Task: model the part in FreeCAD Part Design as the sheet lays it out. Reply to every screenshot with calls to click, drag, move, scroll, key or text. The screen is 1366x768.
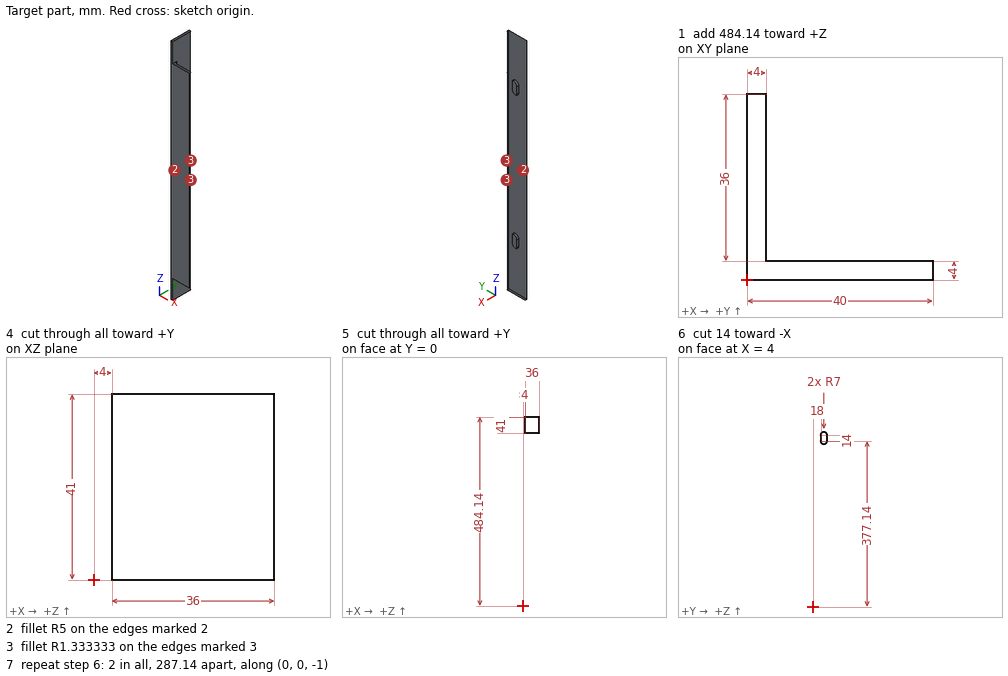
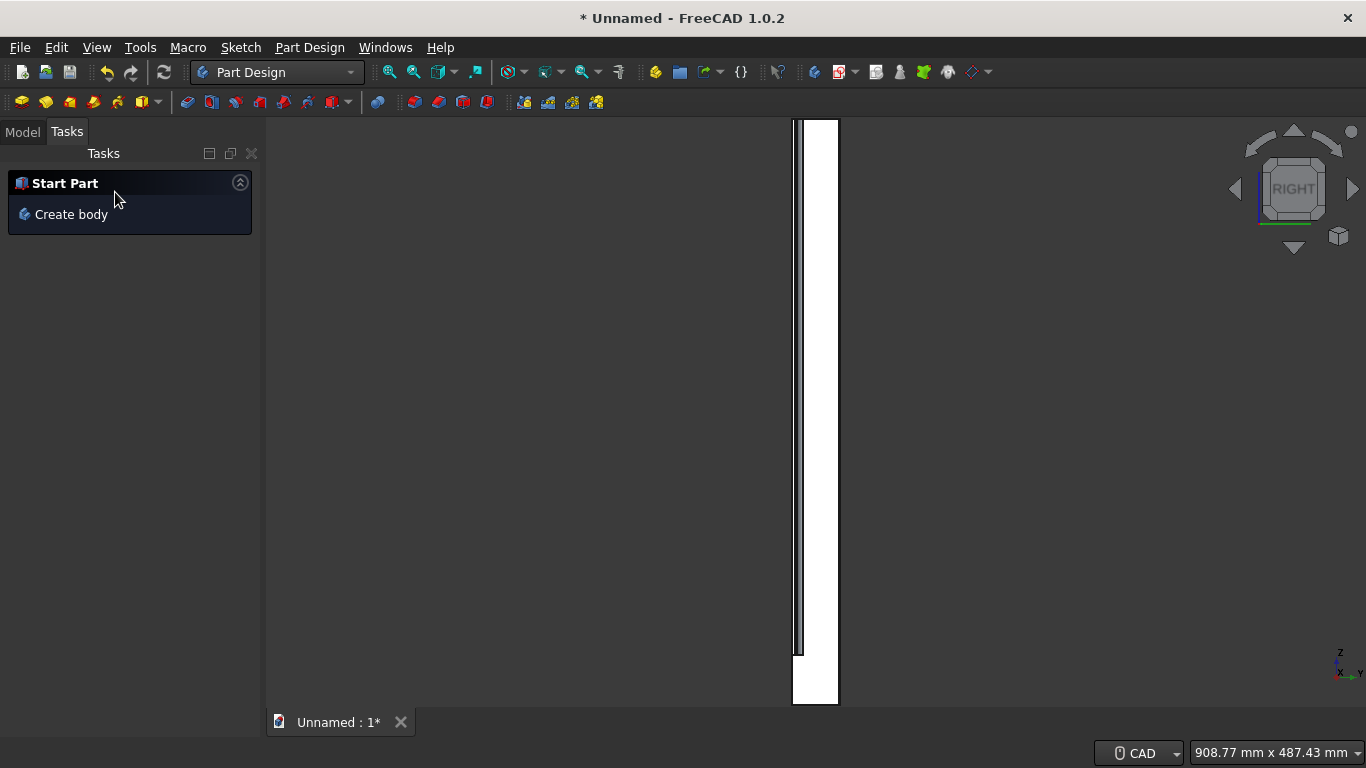
key(0)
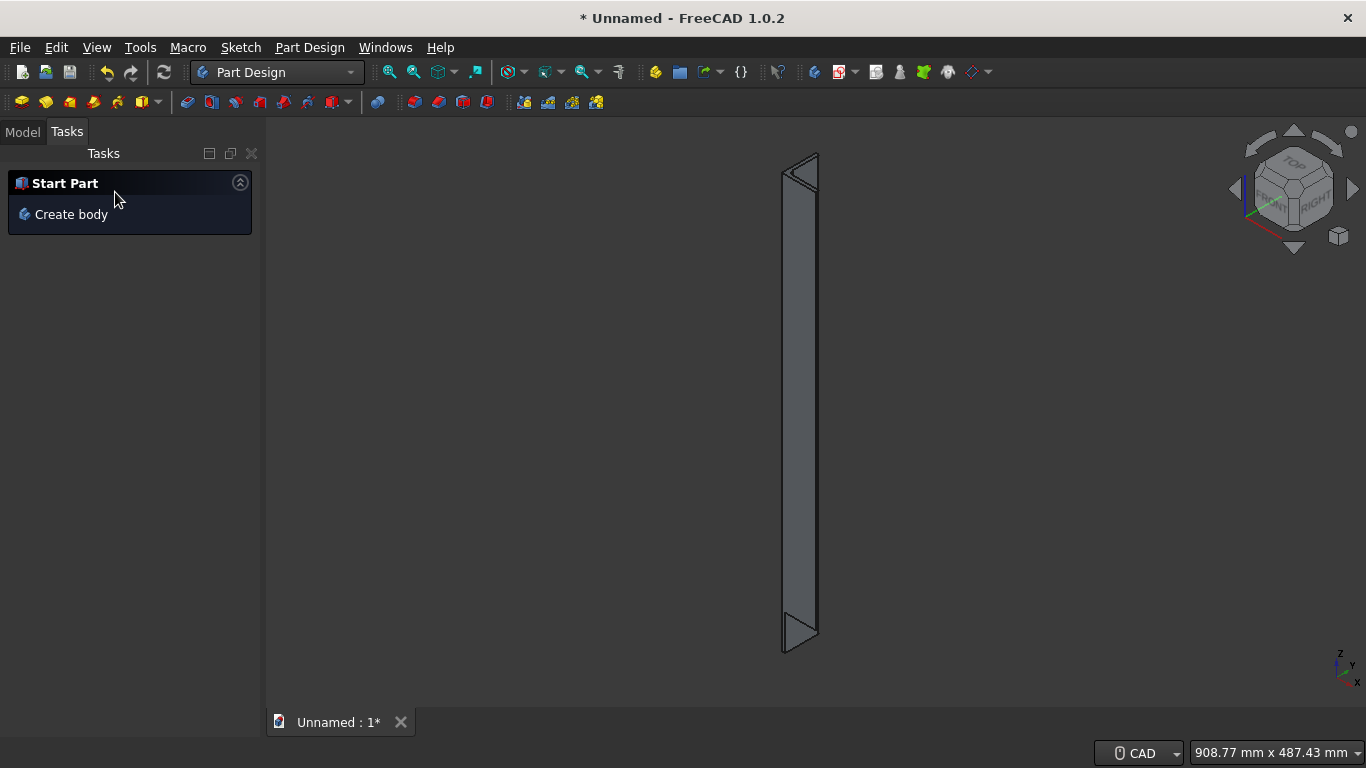
click(799, 216)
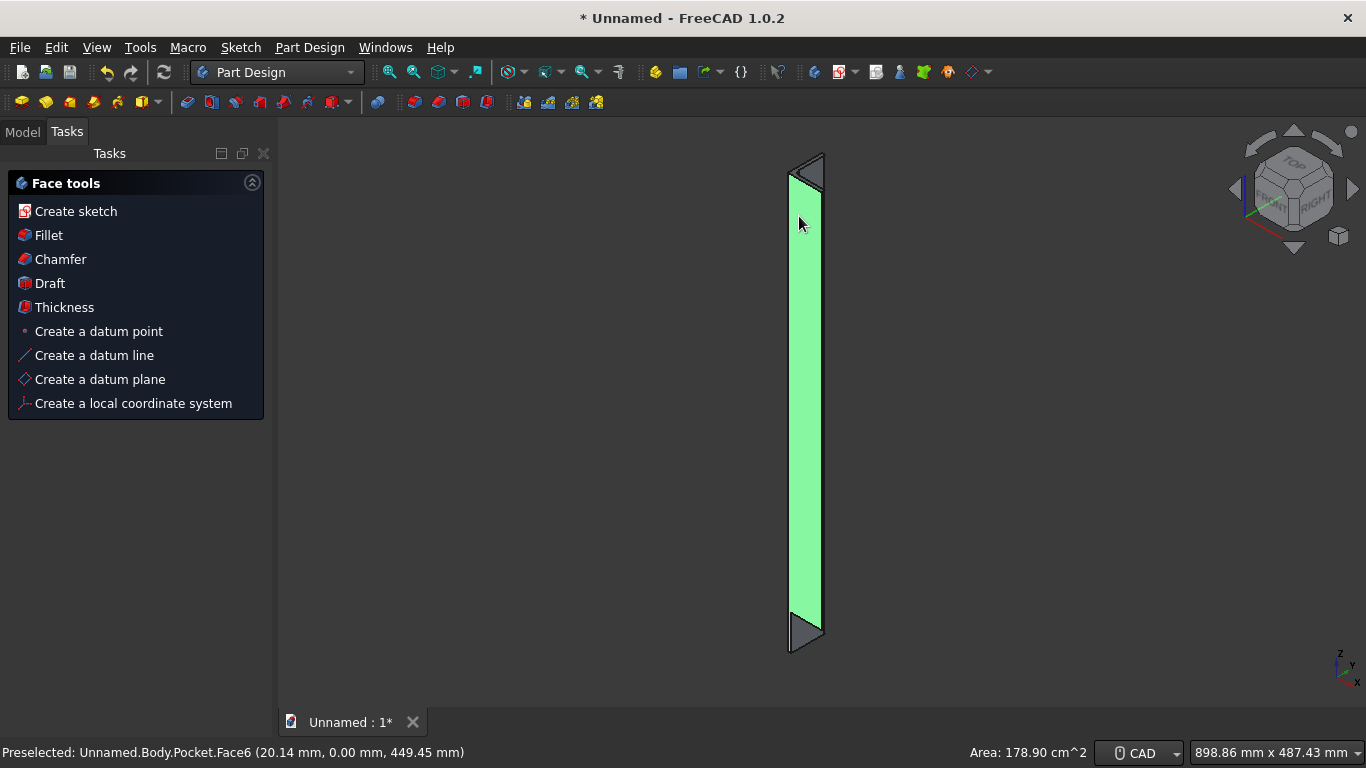
click(840, 72)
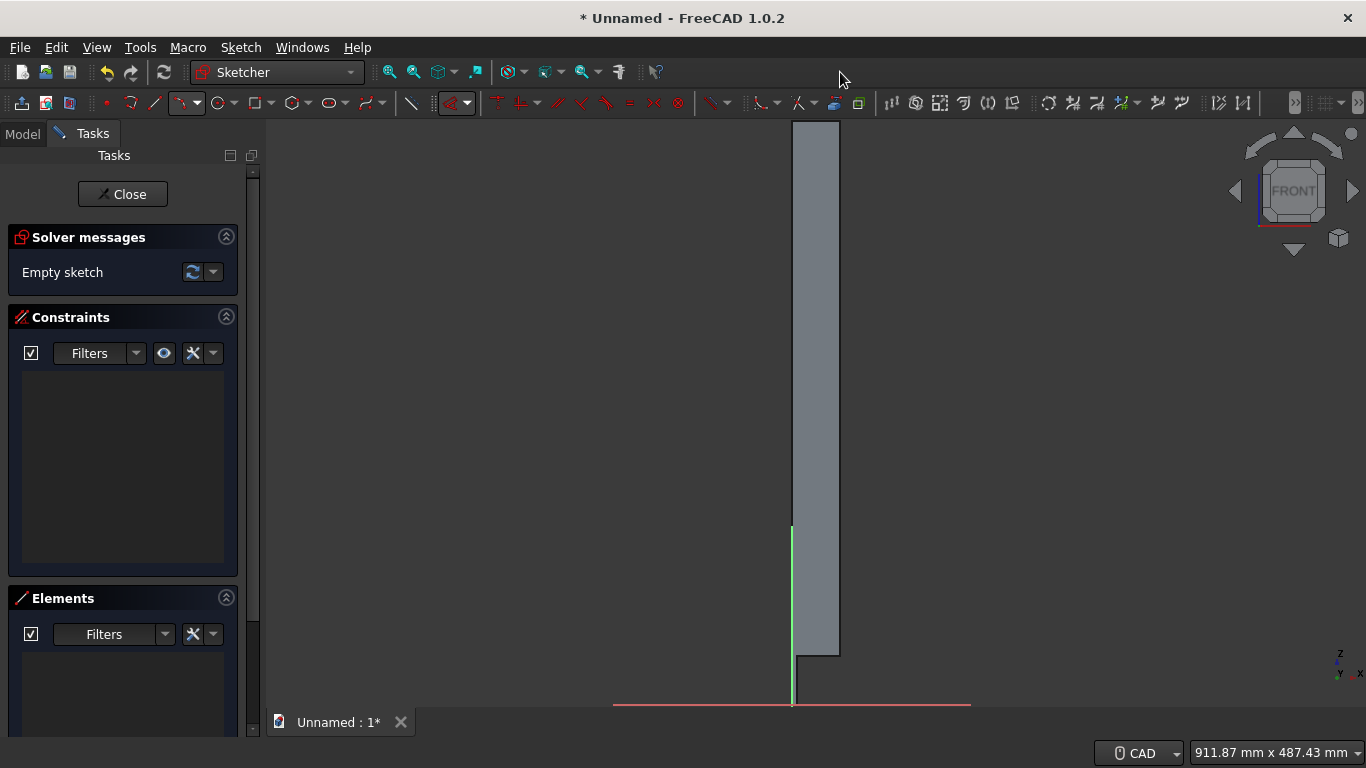
scroll(748, 413, down, 5)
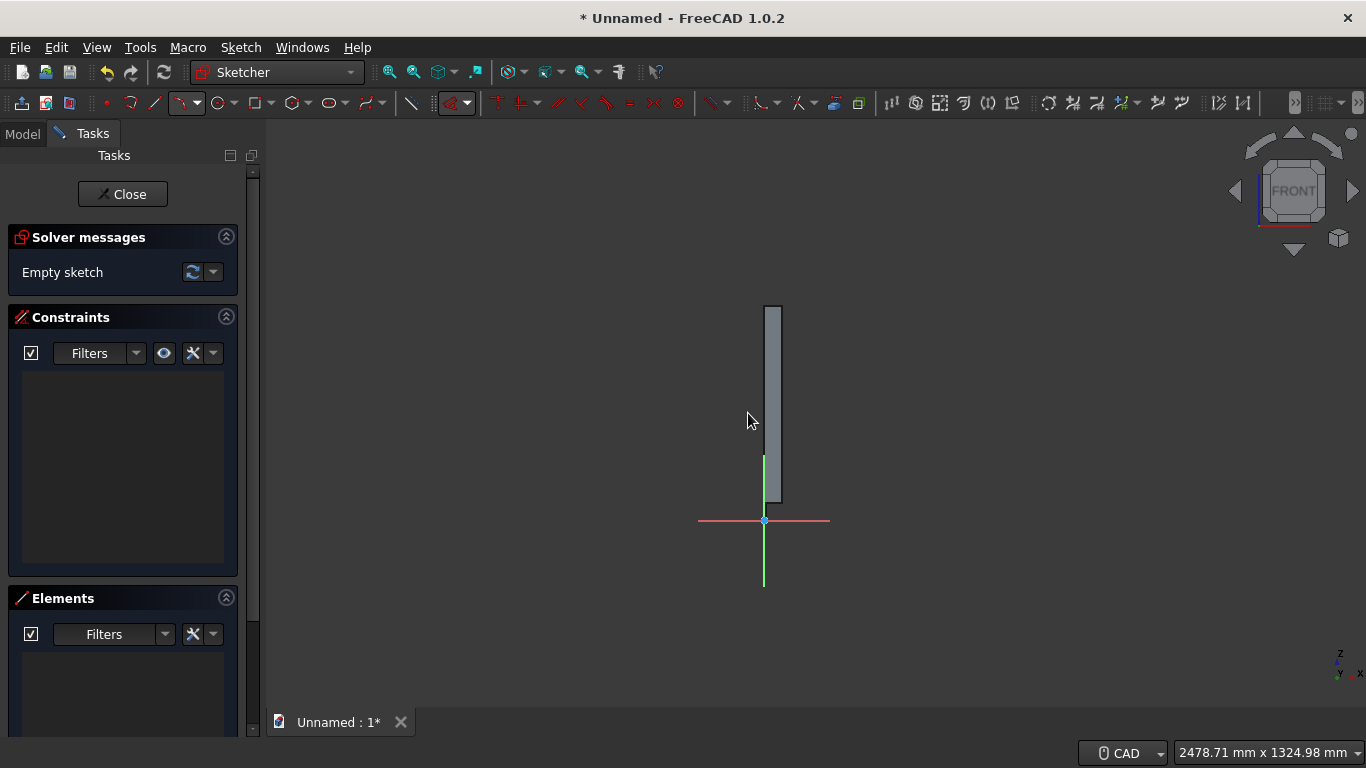
scroll(776, 310, up, 15)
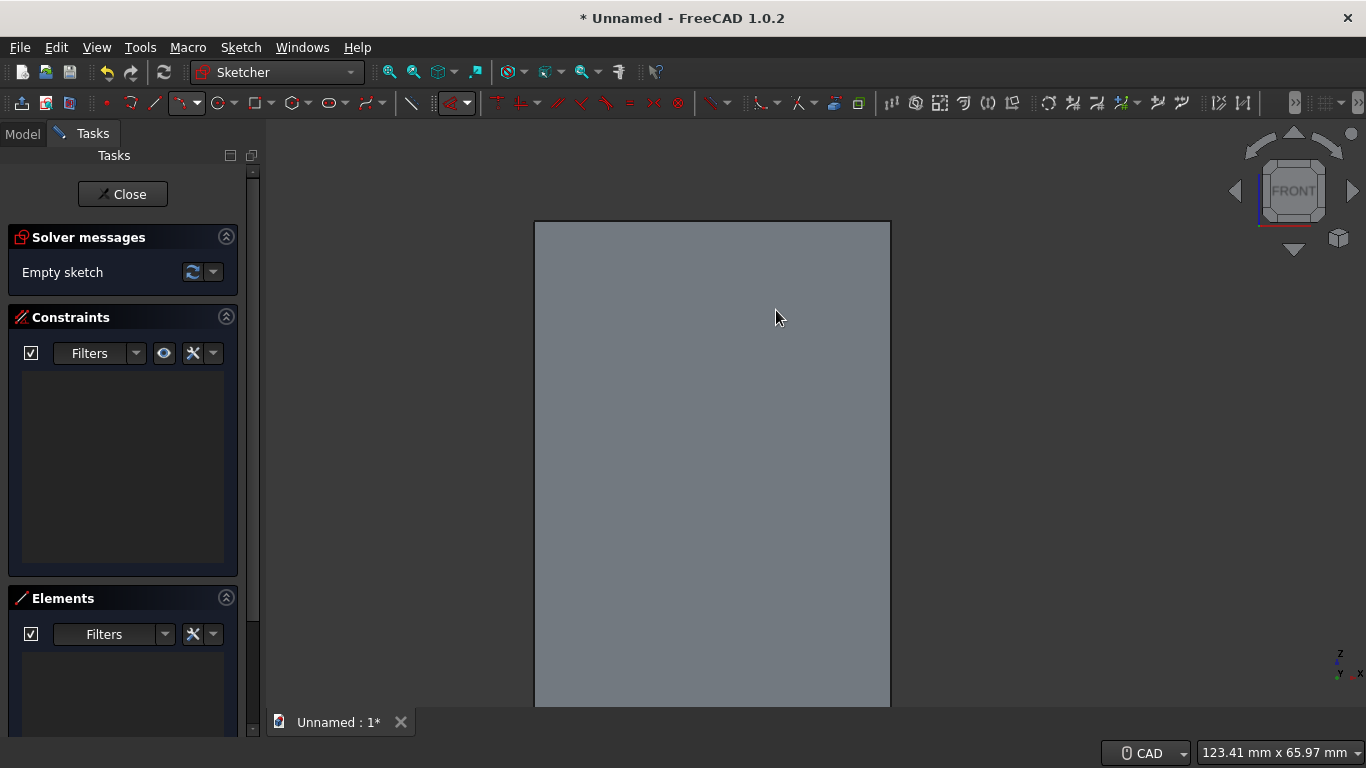
click(256, 104)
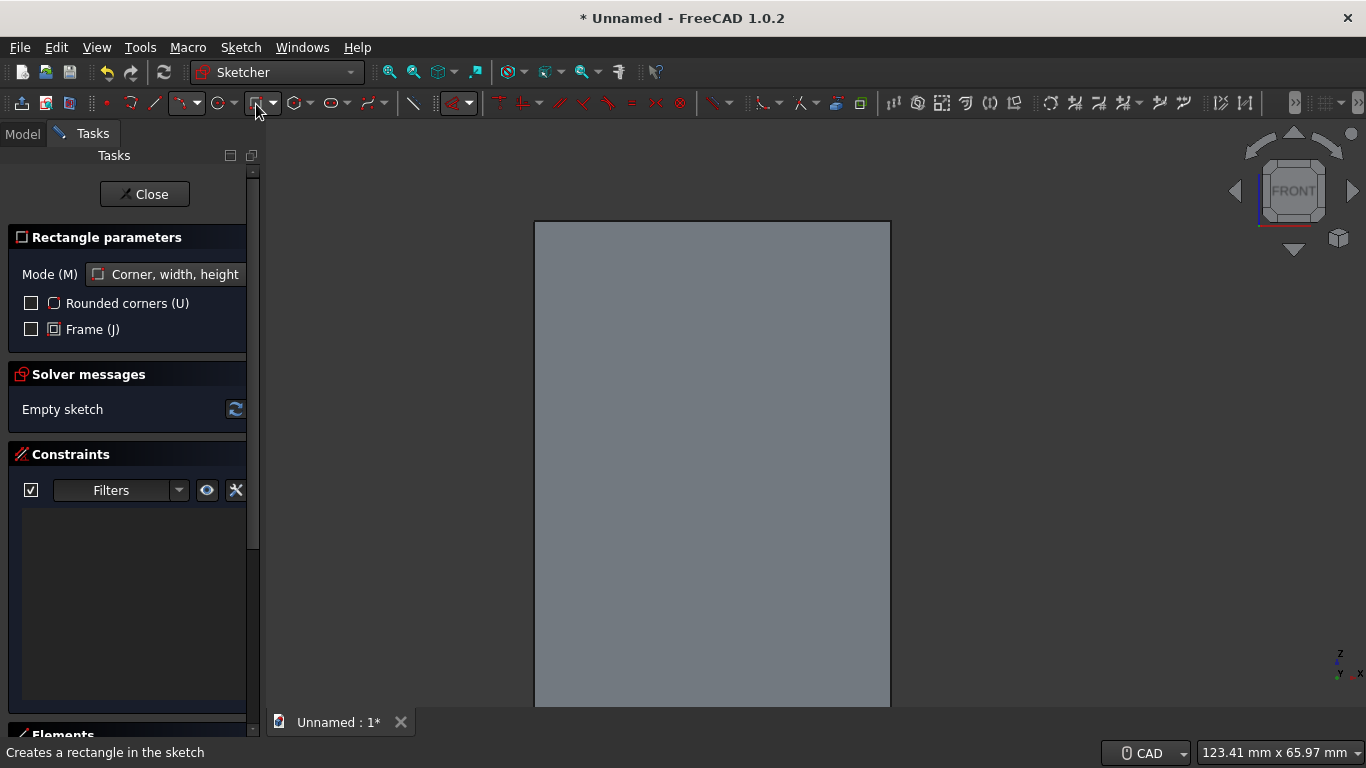
click(570, 221)
click(891, 587)
key(Escape)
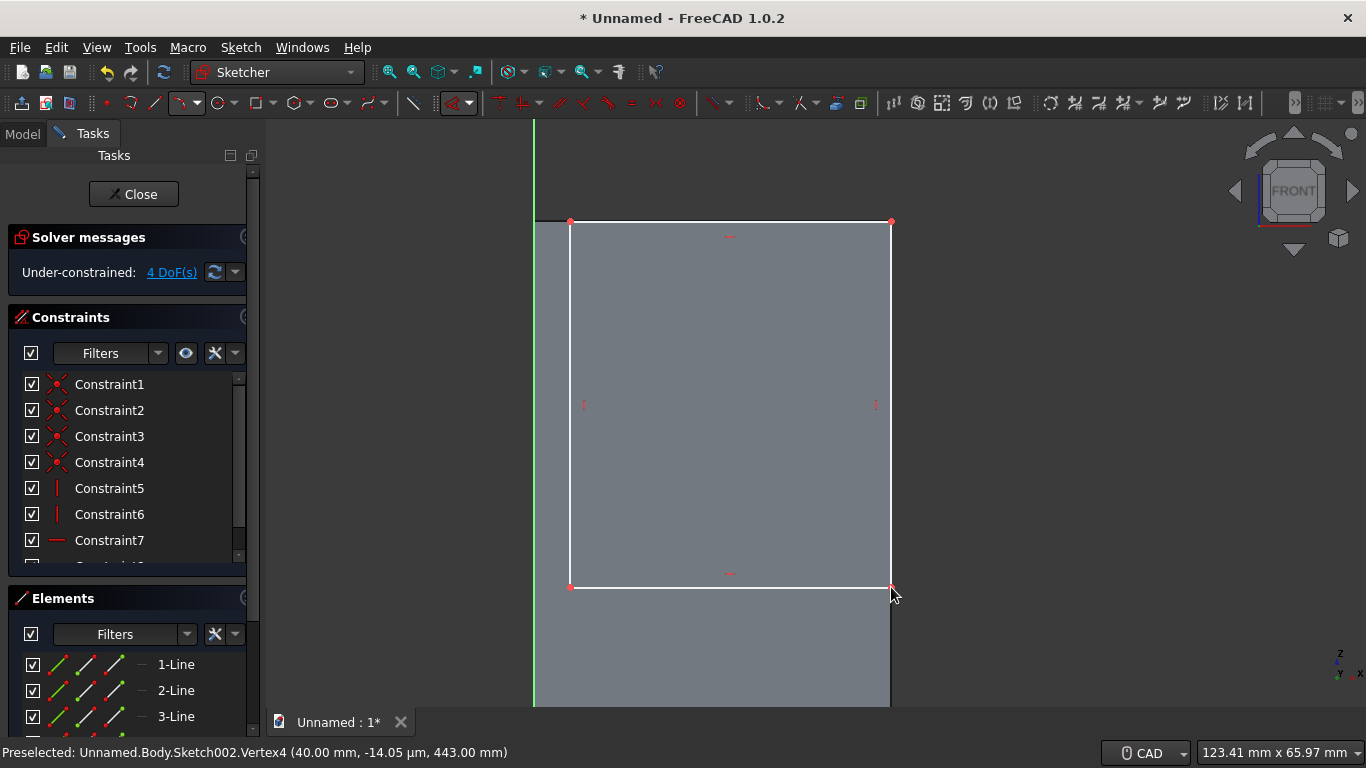
click(570, 332)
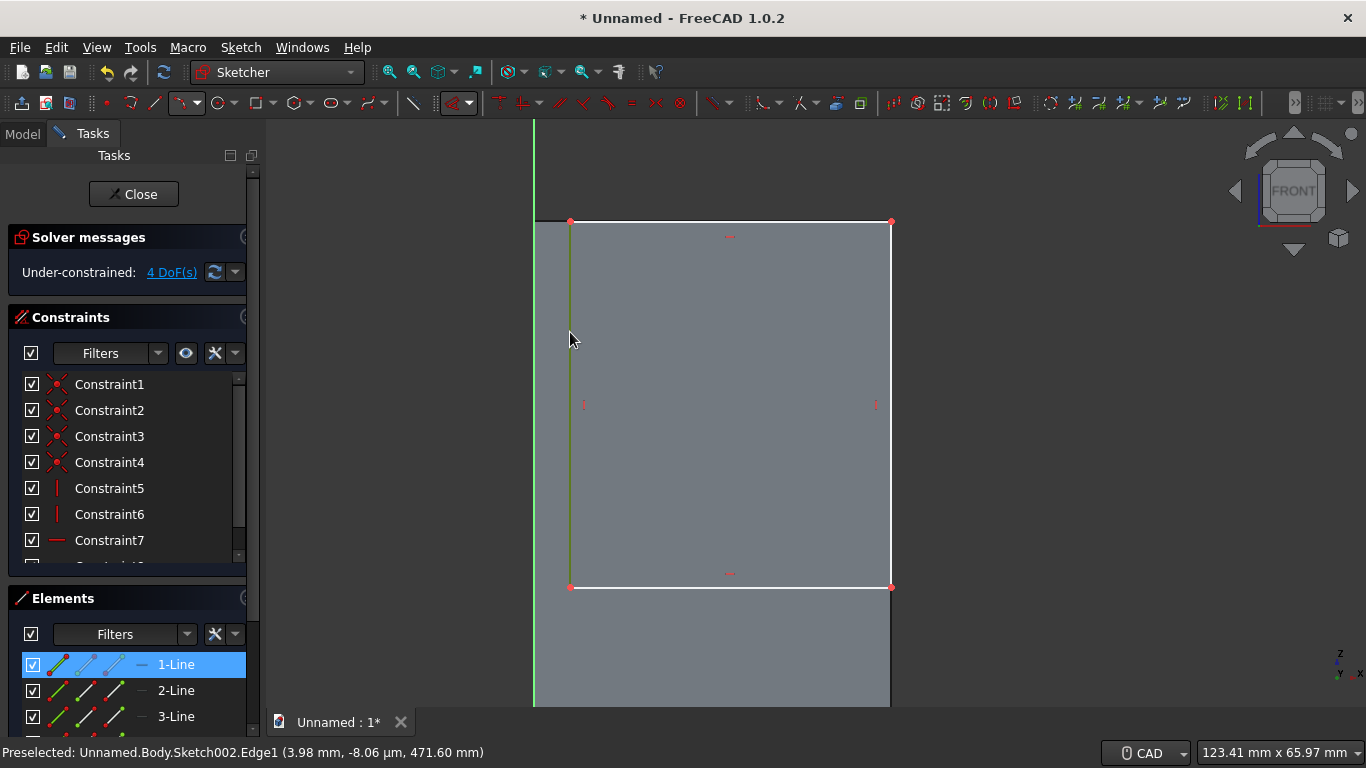
click(472, 104)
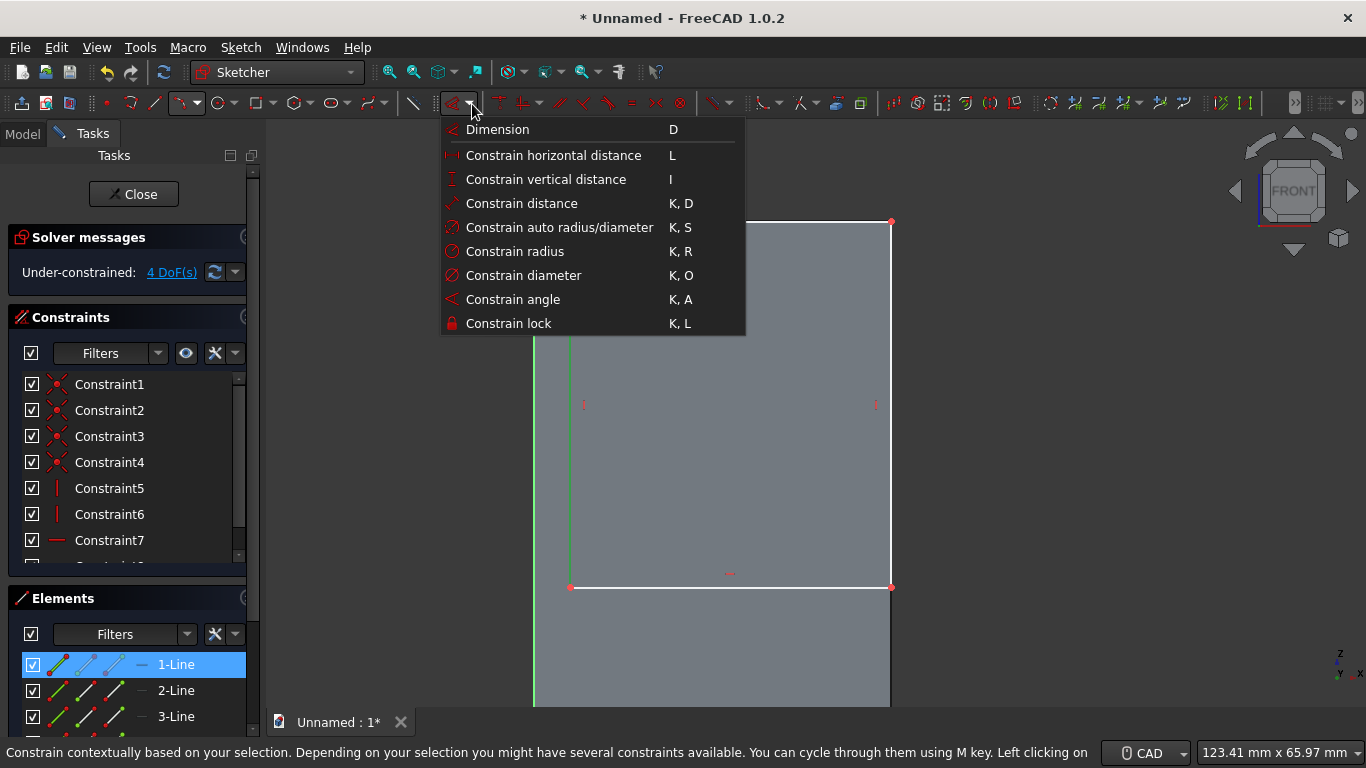
click(593, 179)